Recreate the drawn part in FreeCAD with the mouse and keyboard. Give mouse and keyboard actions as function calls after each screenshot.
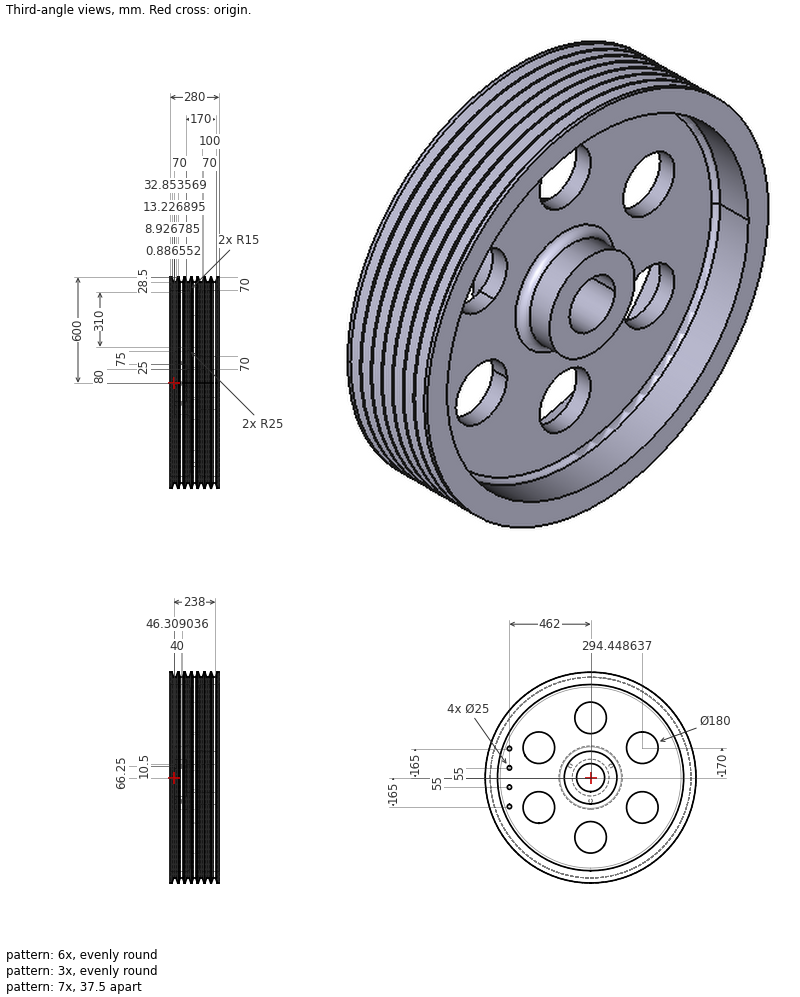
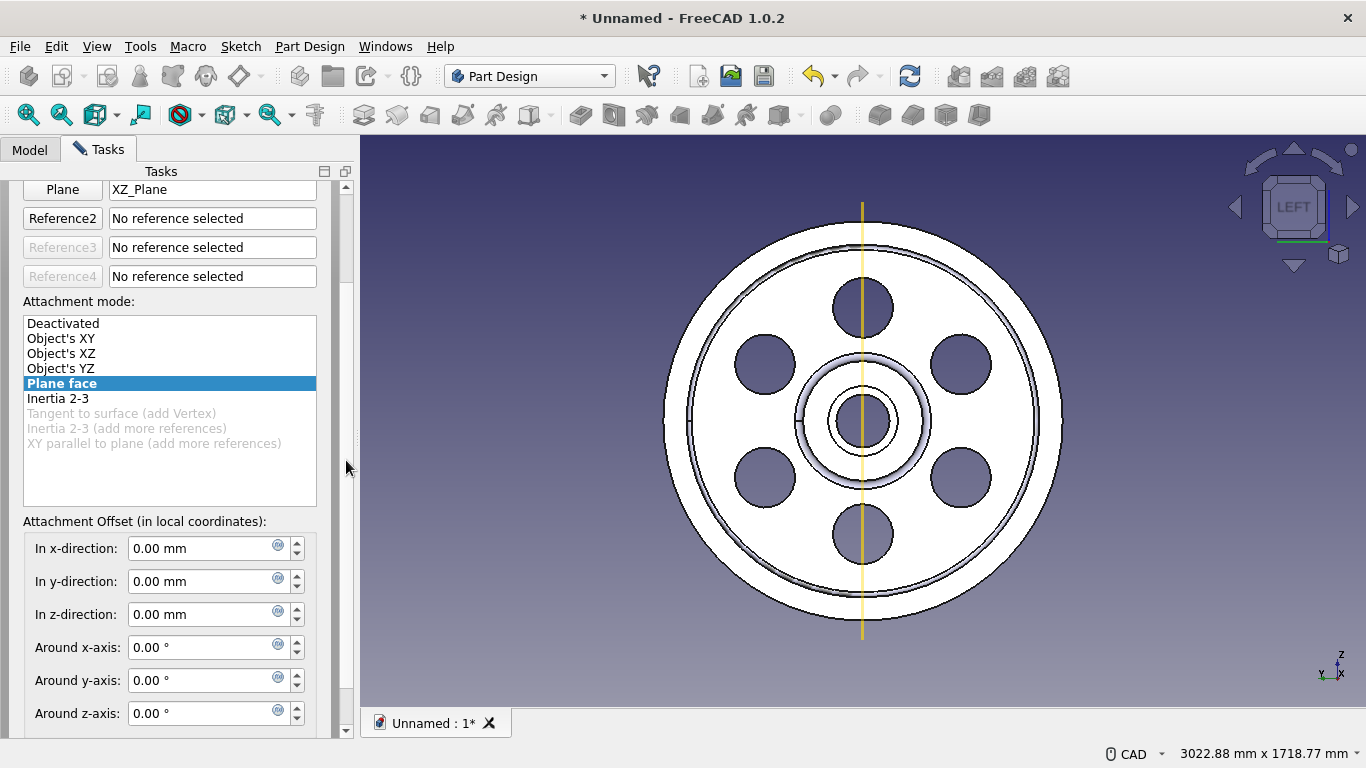
triple_click(210, 614)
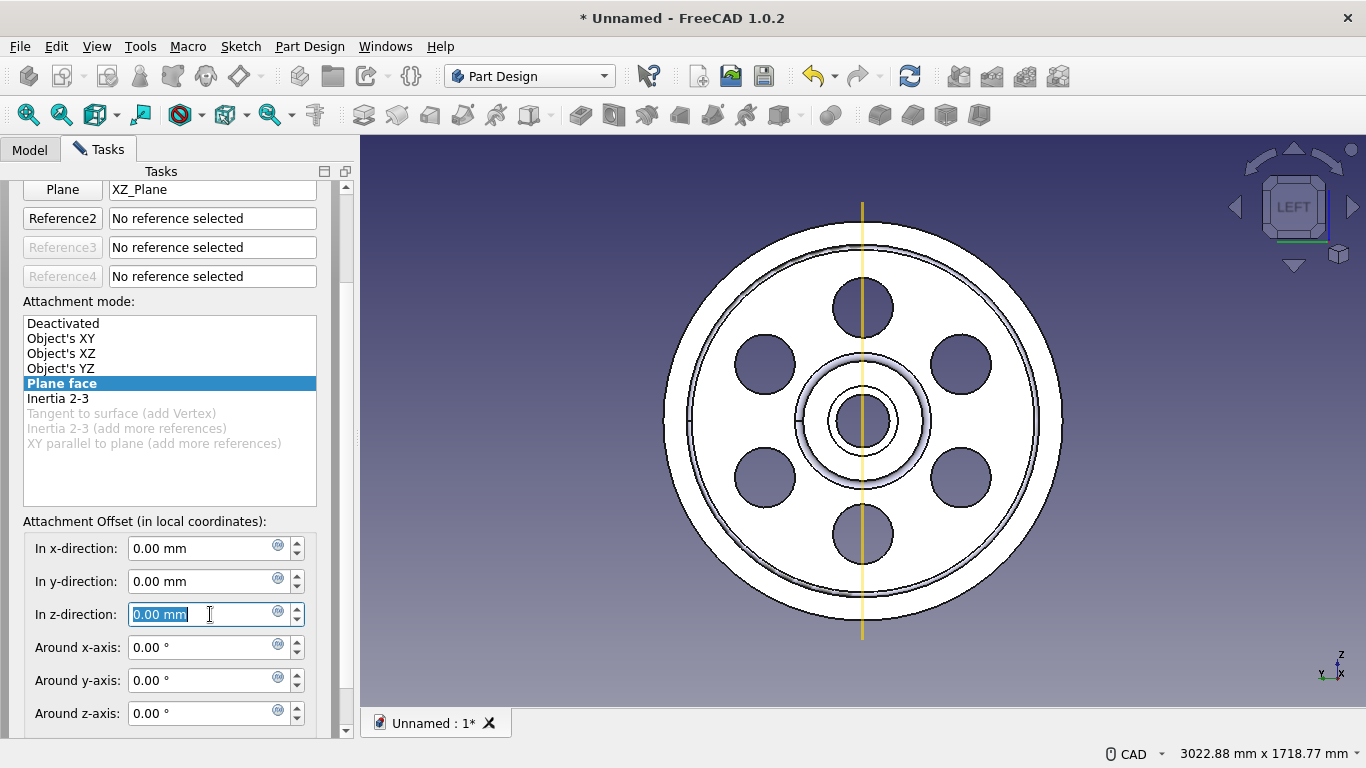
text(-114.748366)
key(Tab)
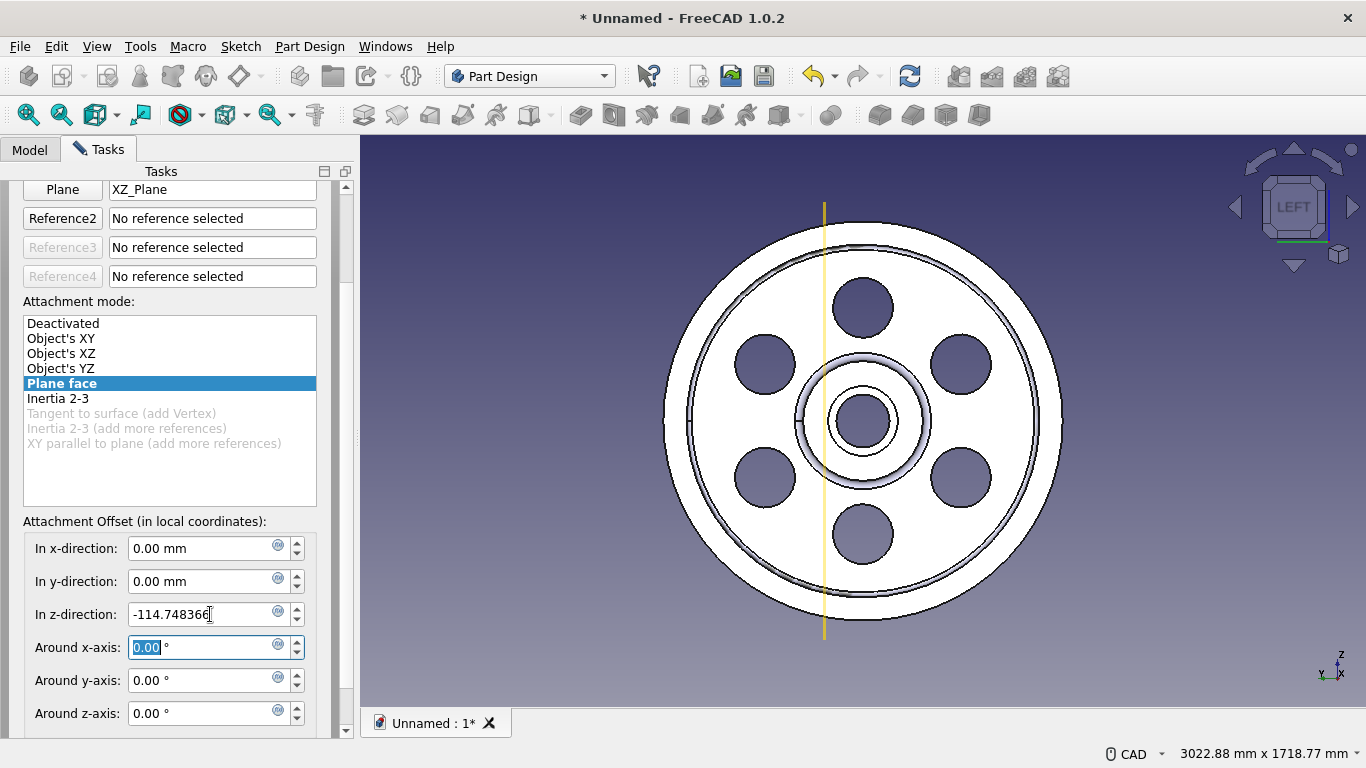
scroll(346, 460, up, 3)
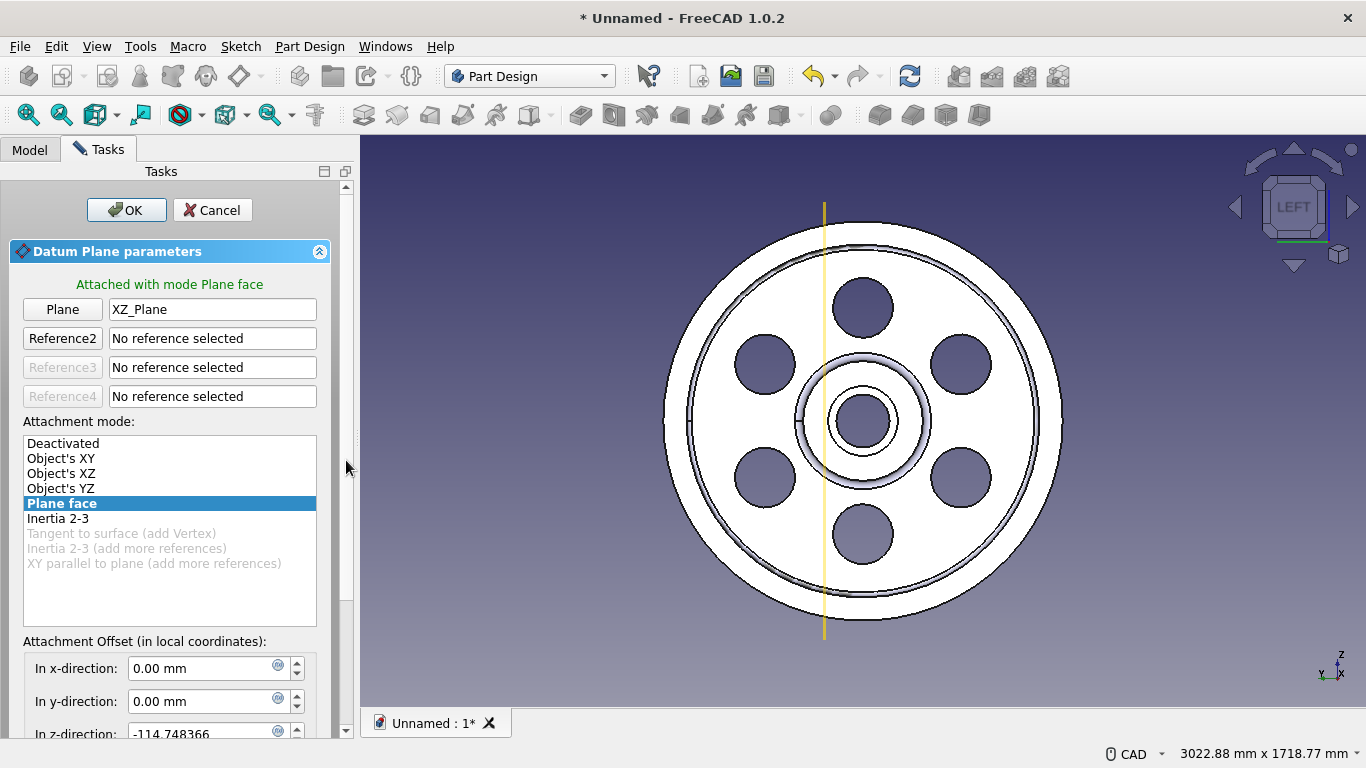
click(127, 210)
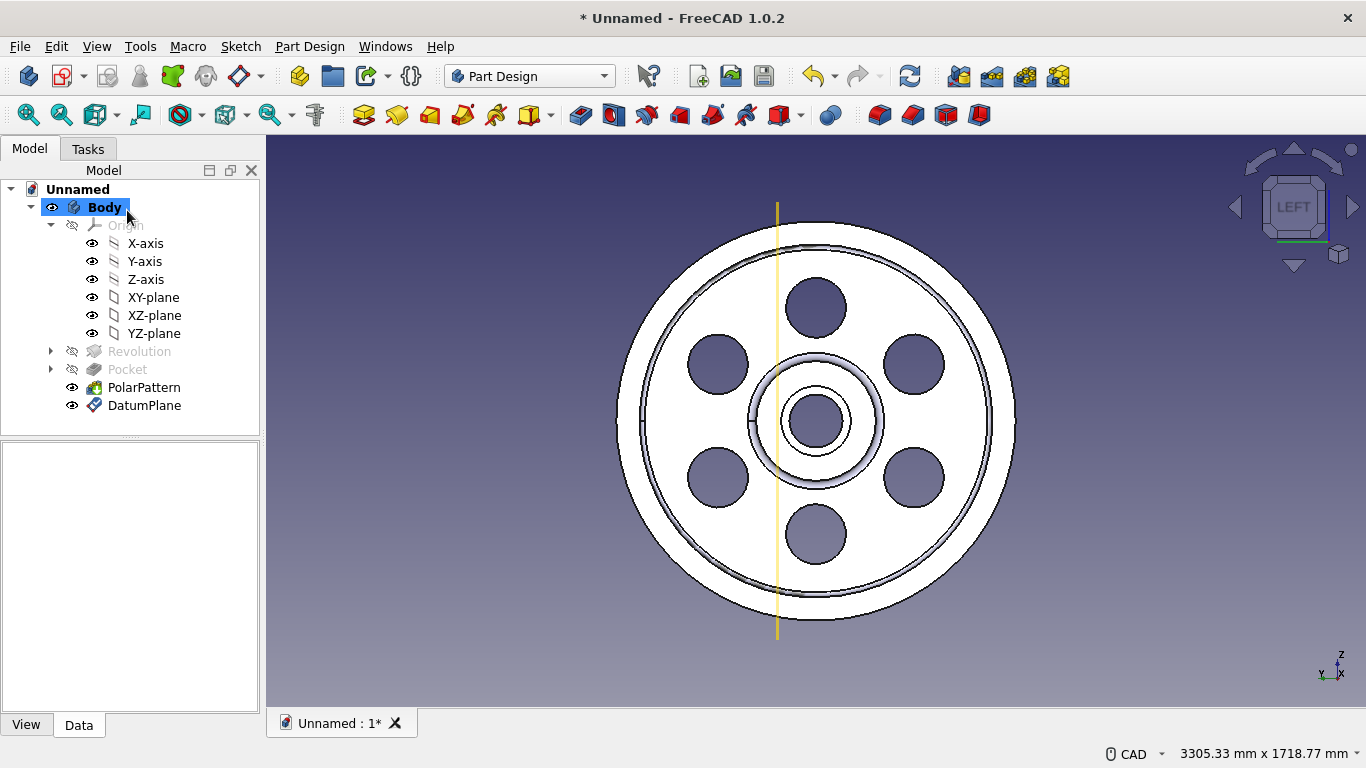
click(117, 405)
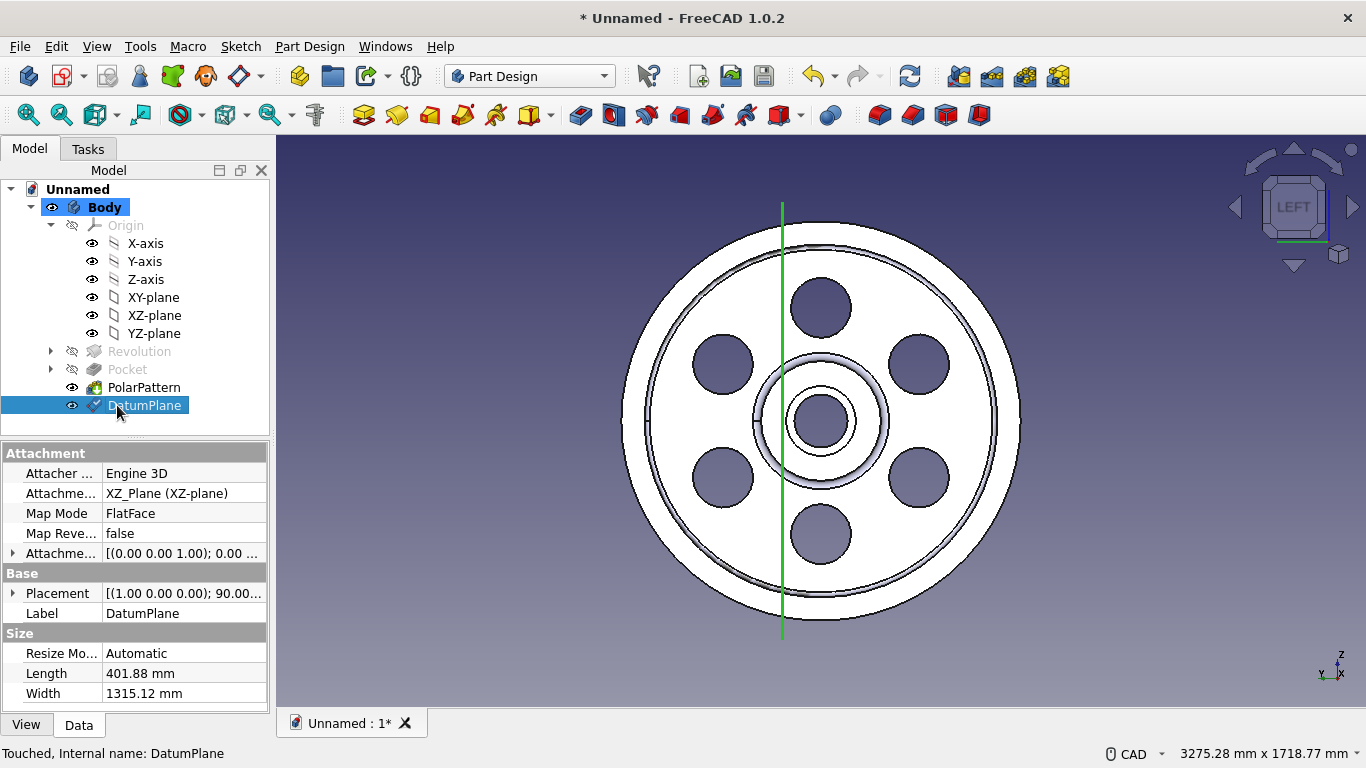
click(62, 76)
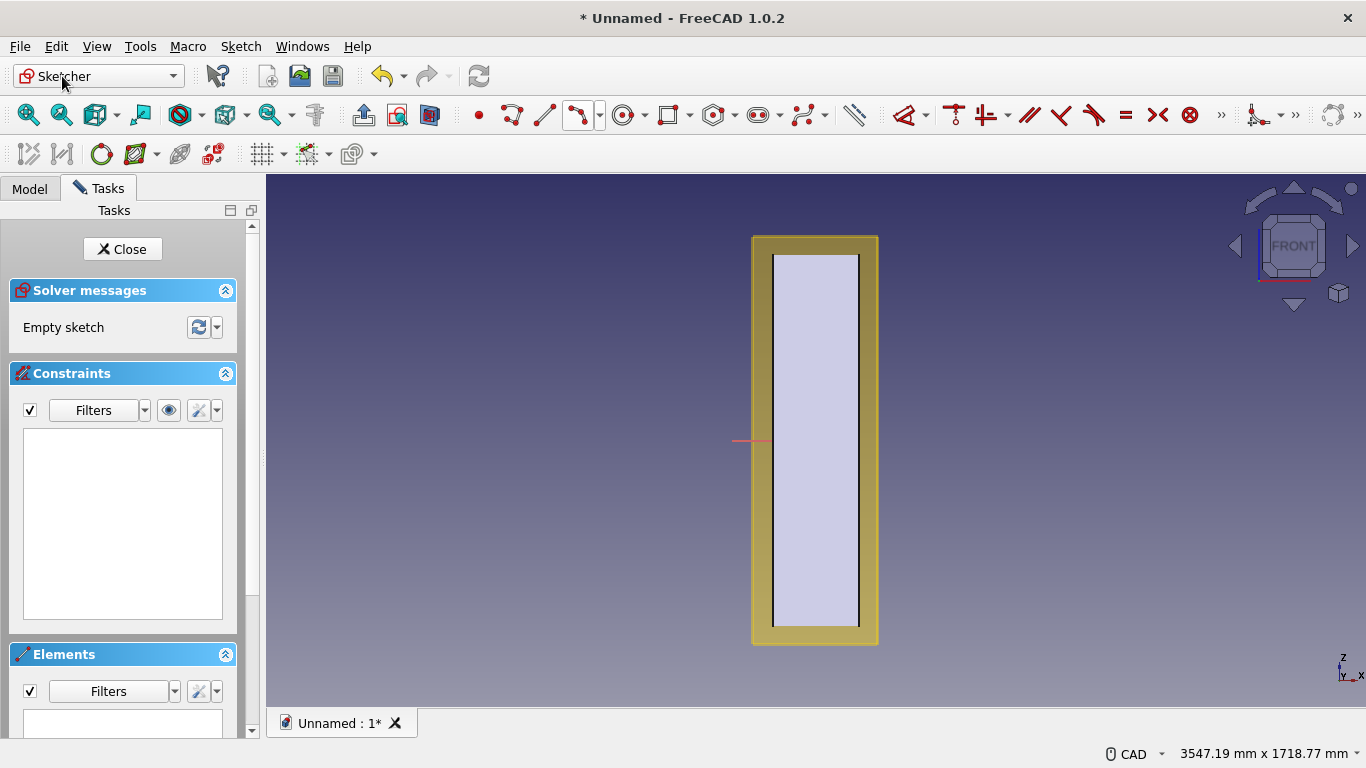
key(q)
key(s)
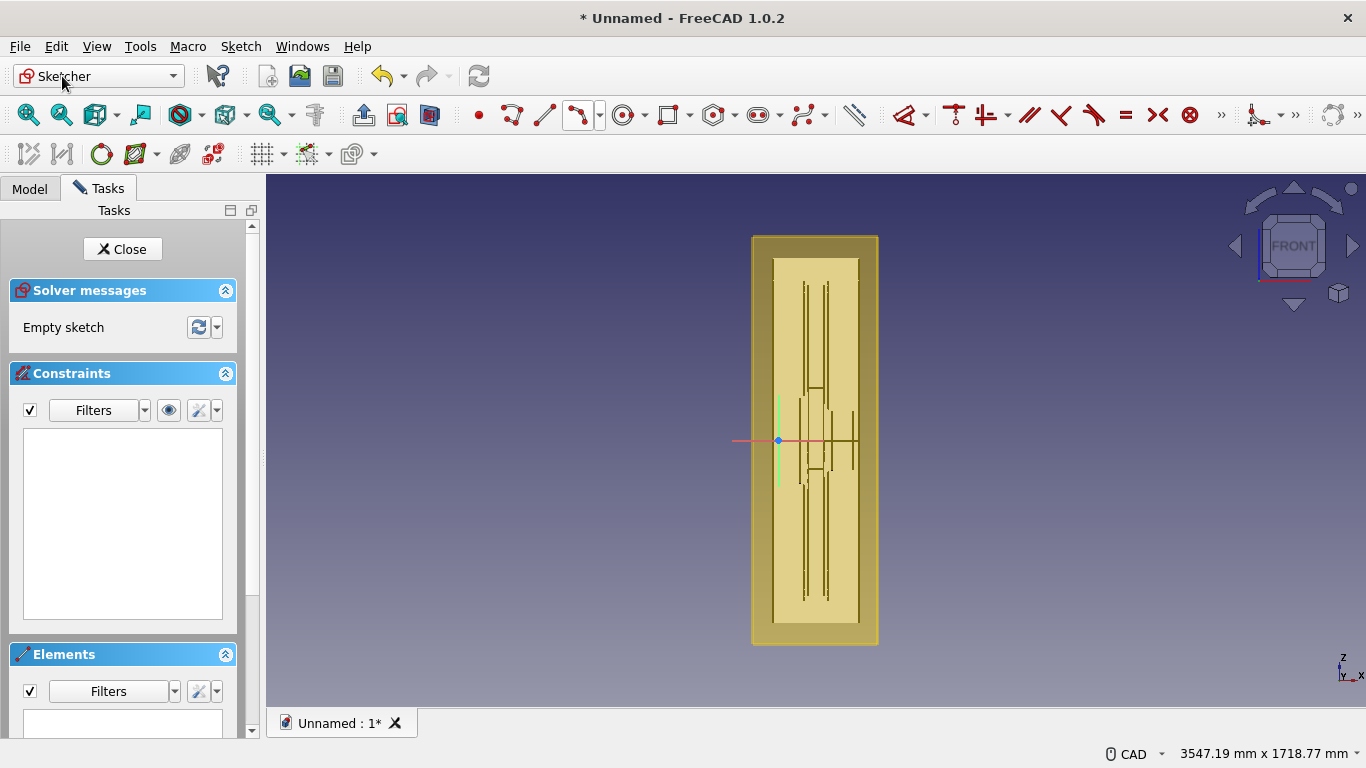
scroll(792, 428, up, 13)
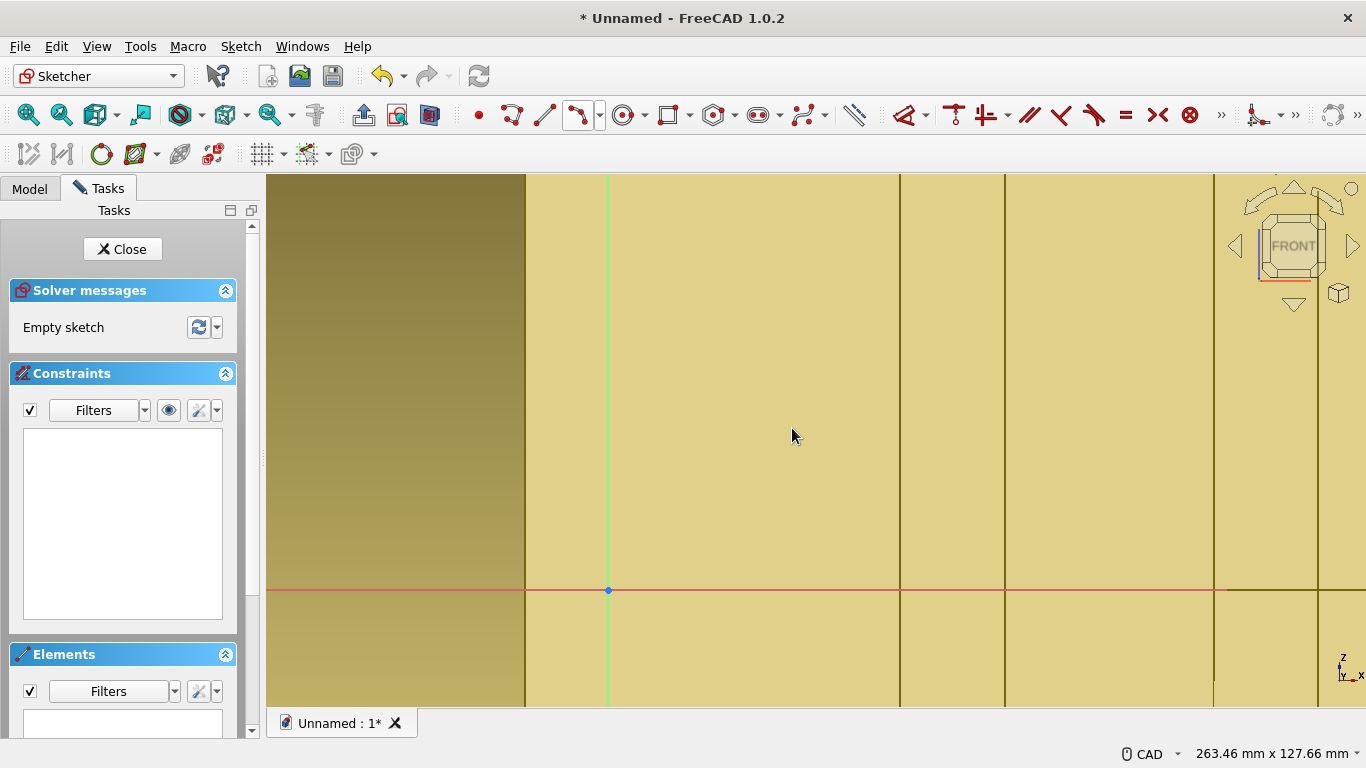
key(g)
key(m)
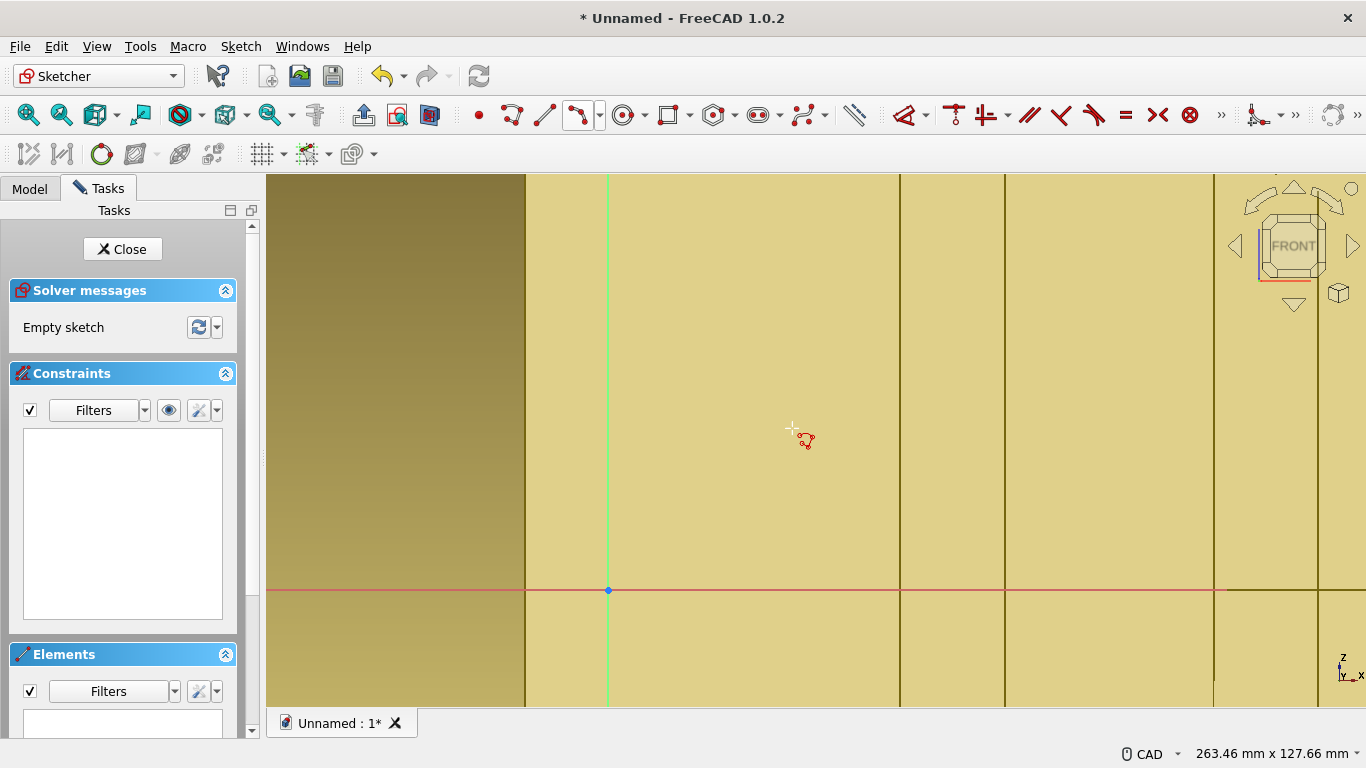
click(608, 314)
click(617, 270)
click(775, 270)
click(801, 314)
click(608, 315)